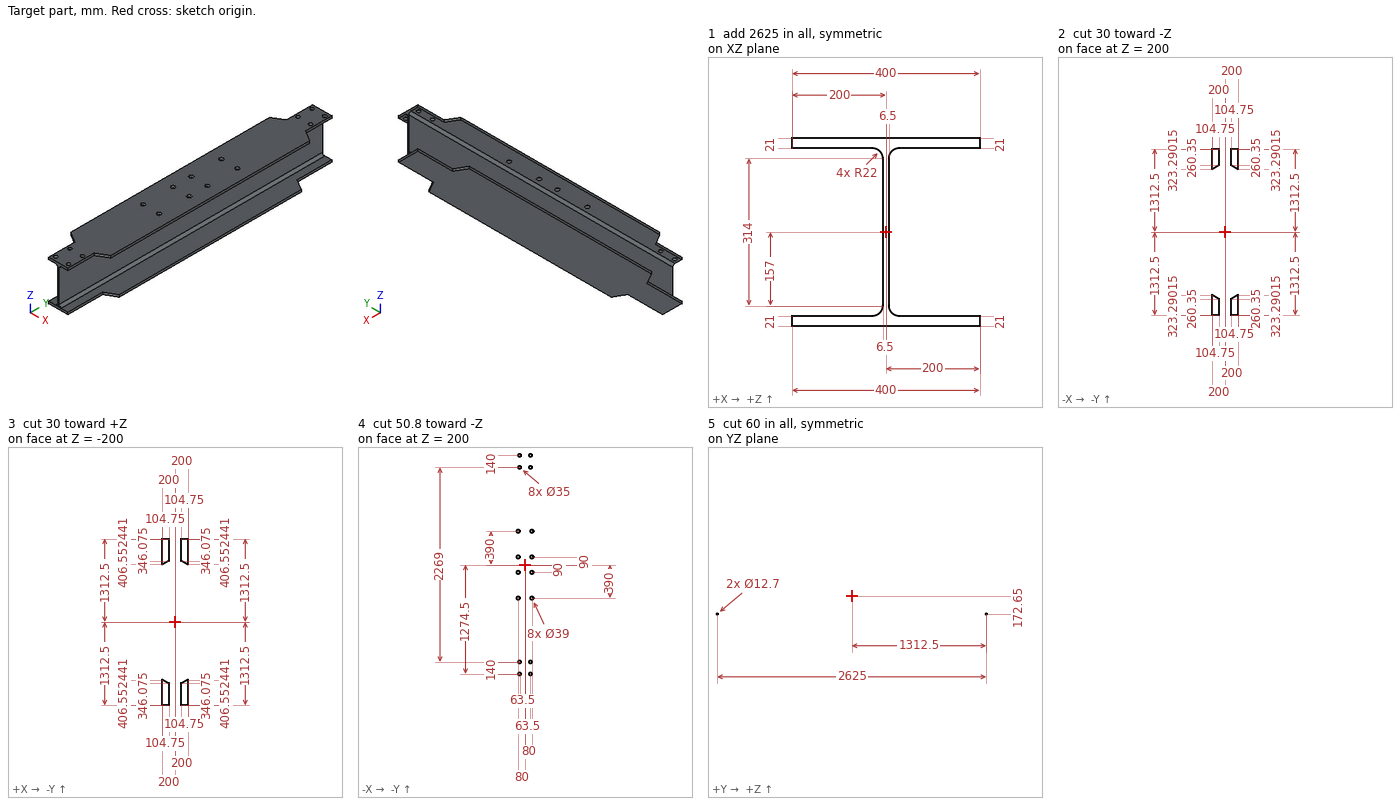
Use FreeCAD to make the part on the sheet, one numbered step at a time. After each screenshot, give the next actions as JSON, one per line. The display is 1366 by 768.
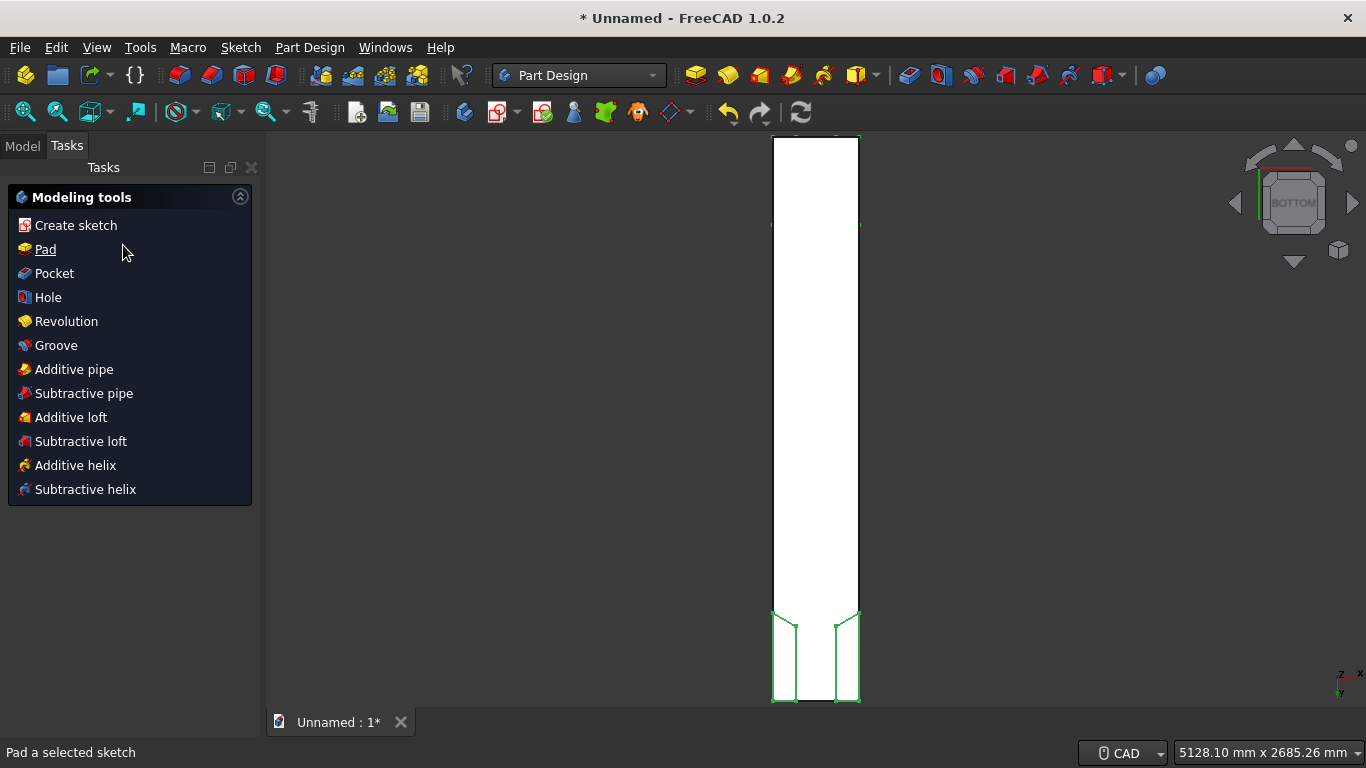
{"action": "left_click", "coordinate": [910, 76]}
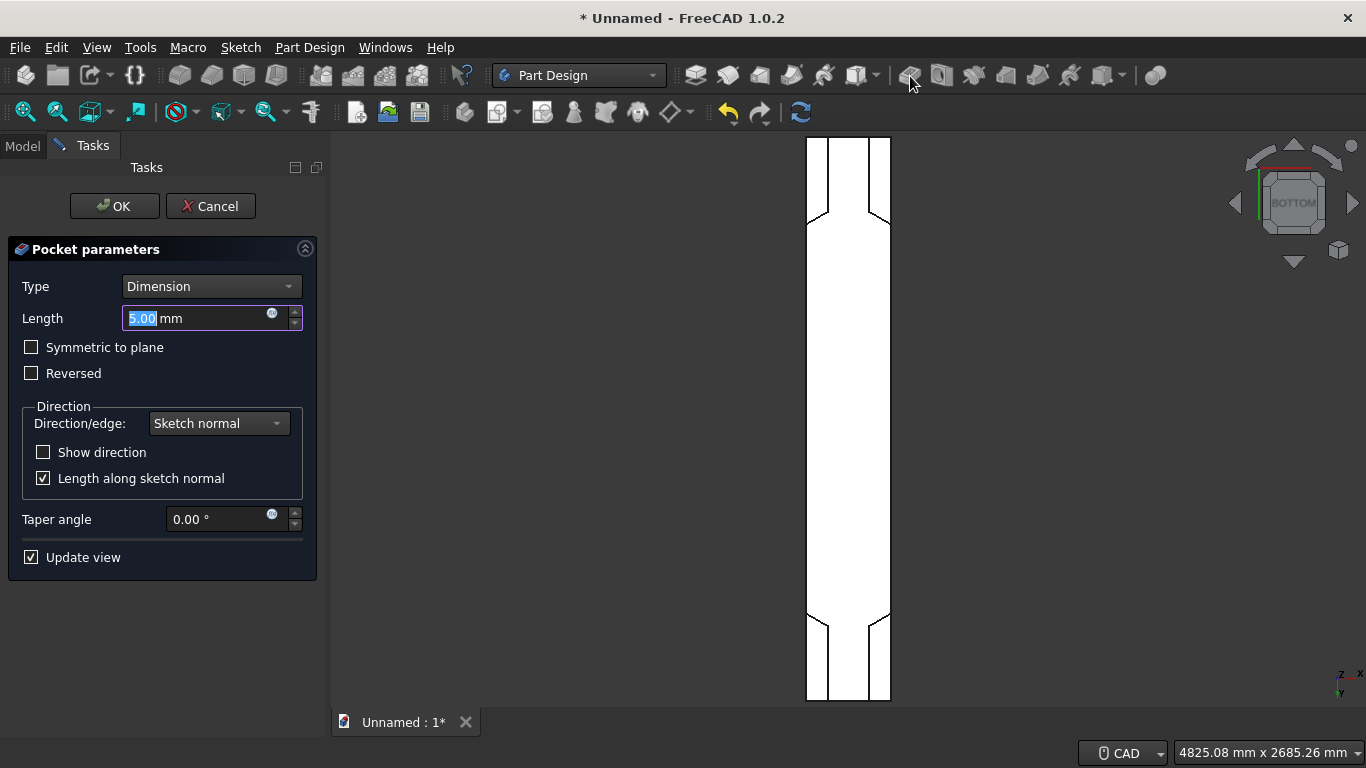
{"action": "type", "text": "30"}
{"action": "key", "text": "Tab"}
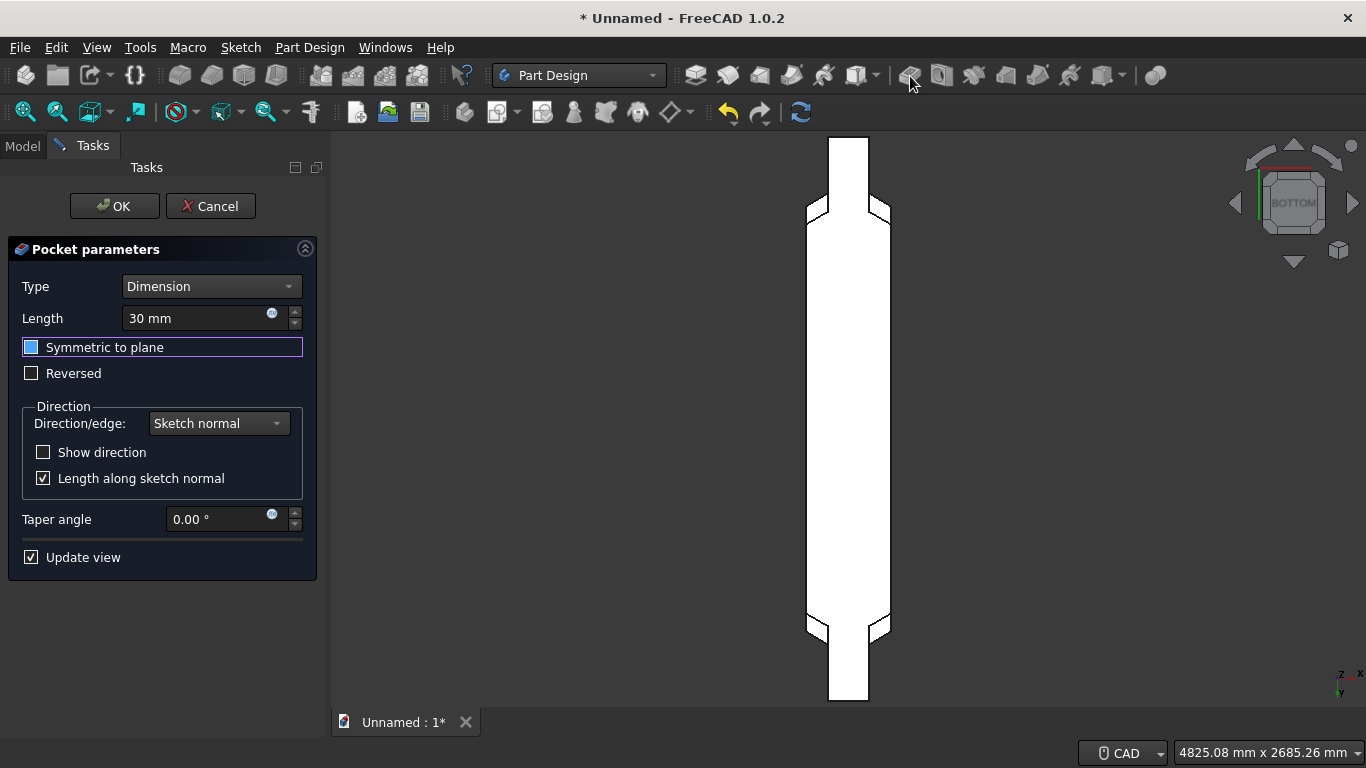
{"action": "left_click", "coordinate": [115, 206]}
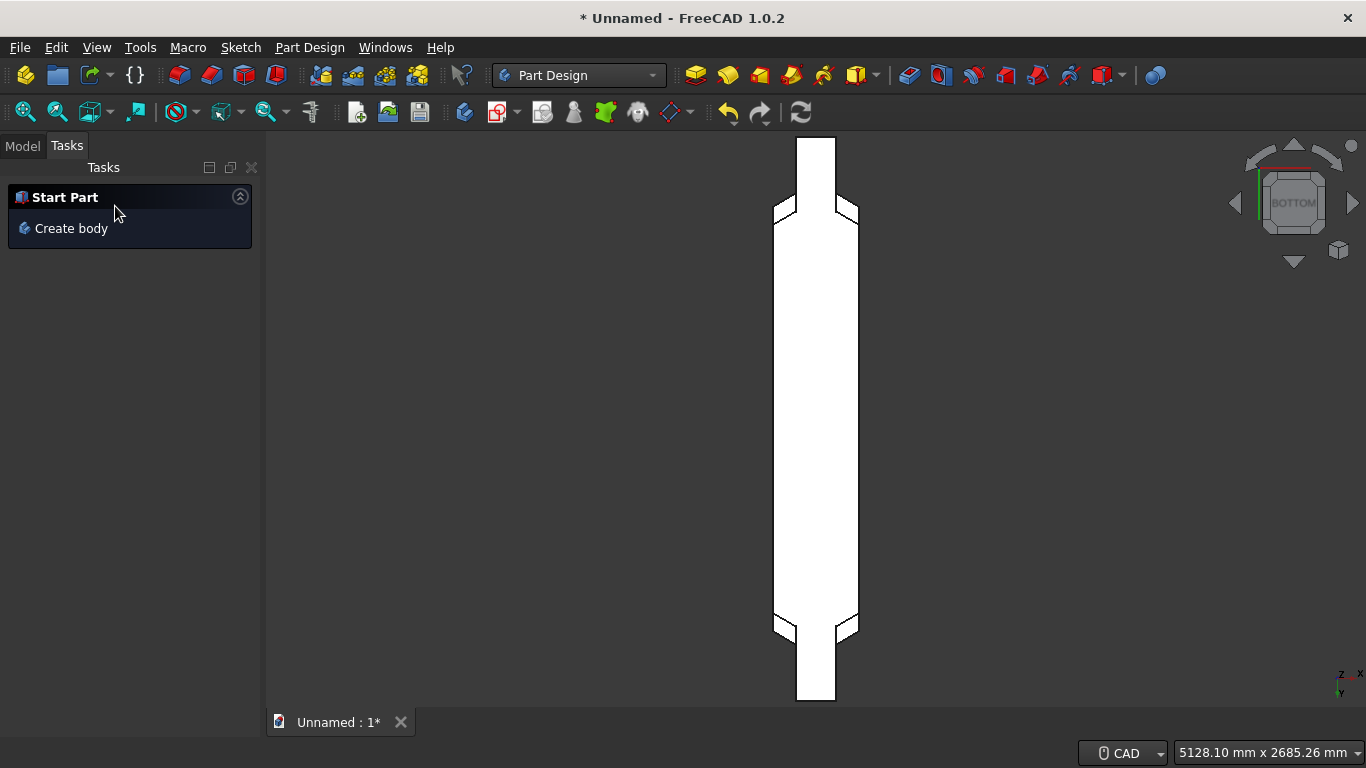
{"action": "key", "text": "0"}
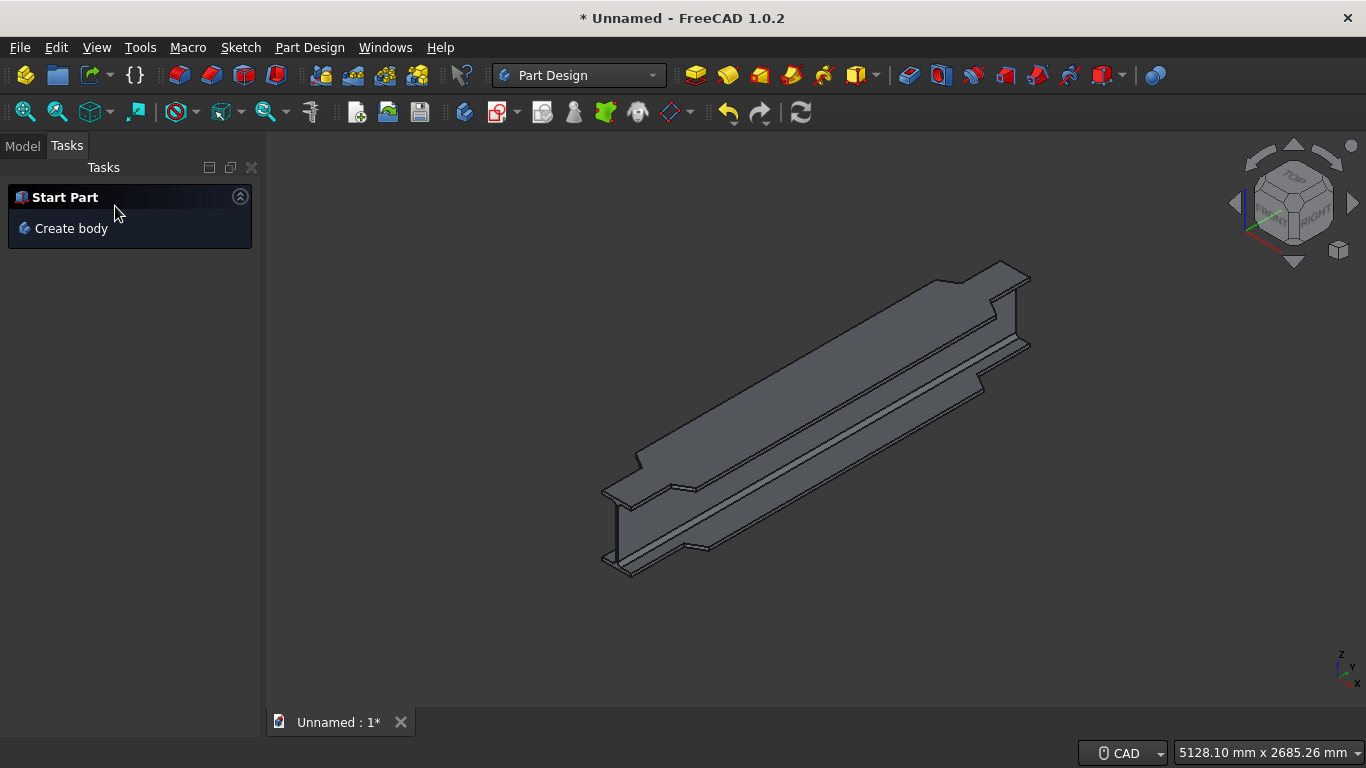
{"action": "left_click", "coordinate": [930, 317]}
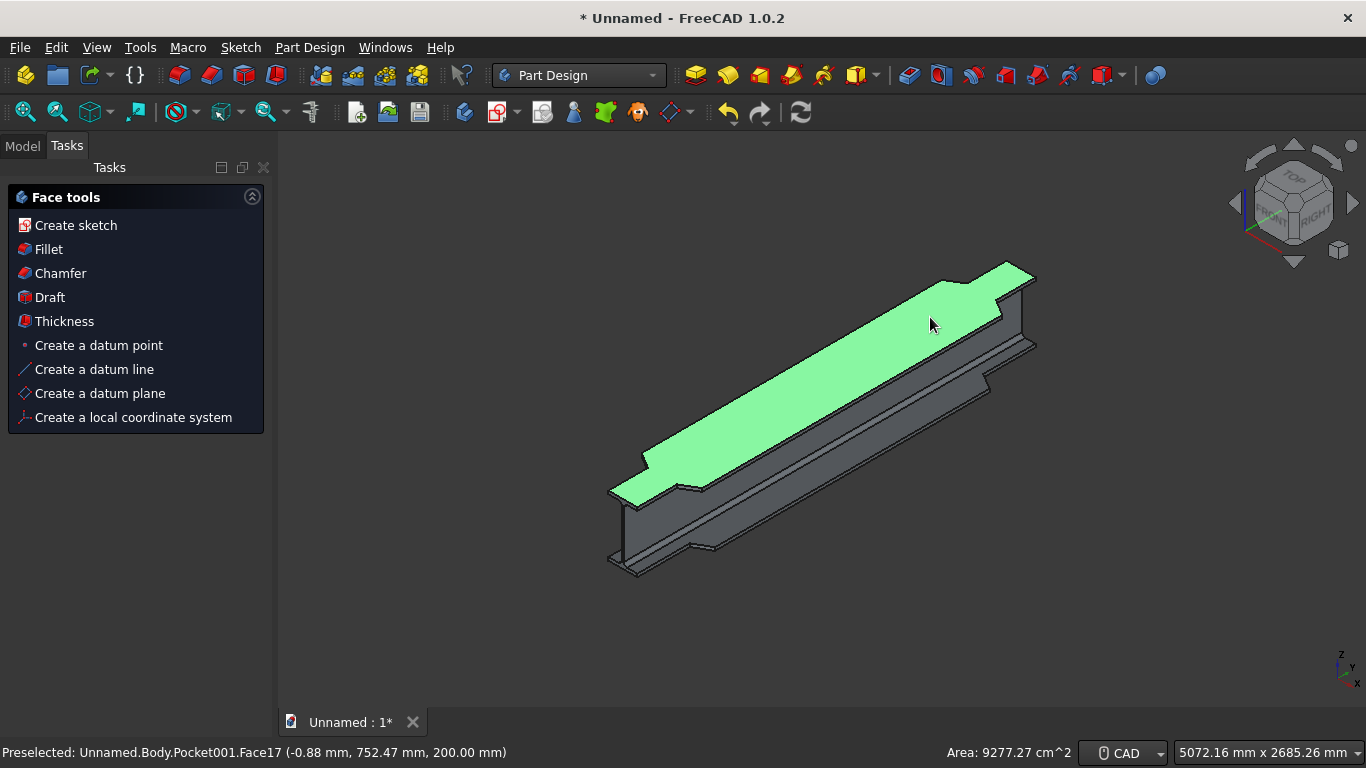
{"action": "left_click", "coordinate": [498, 112]}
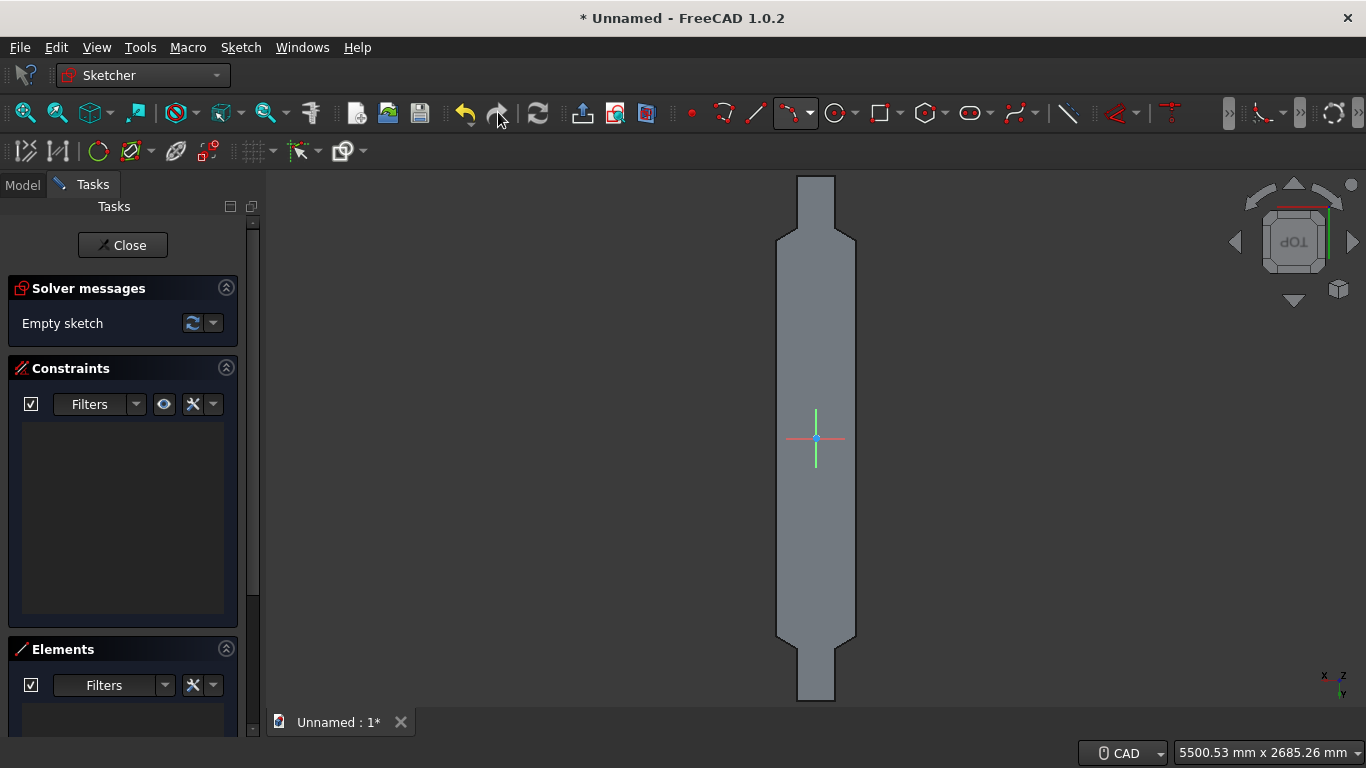
{"action": "scroll", "coordinate": [608, 438], "scroll_direction": "down", "scroll_amount": 2}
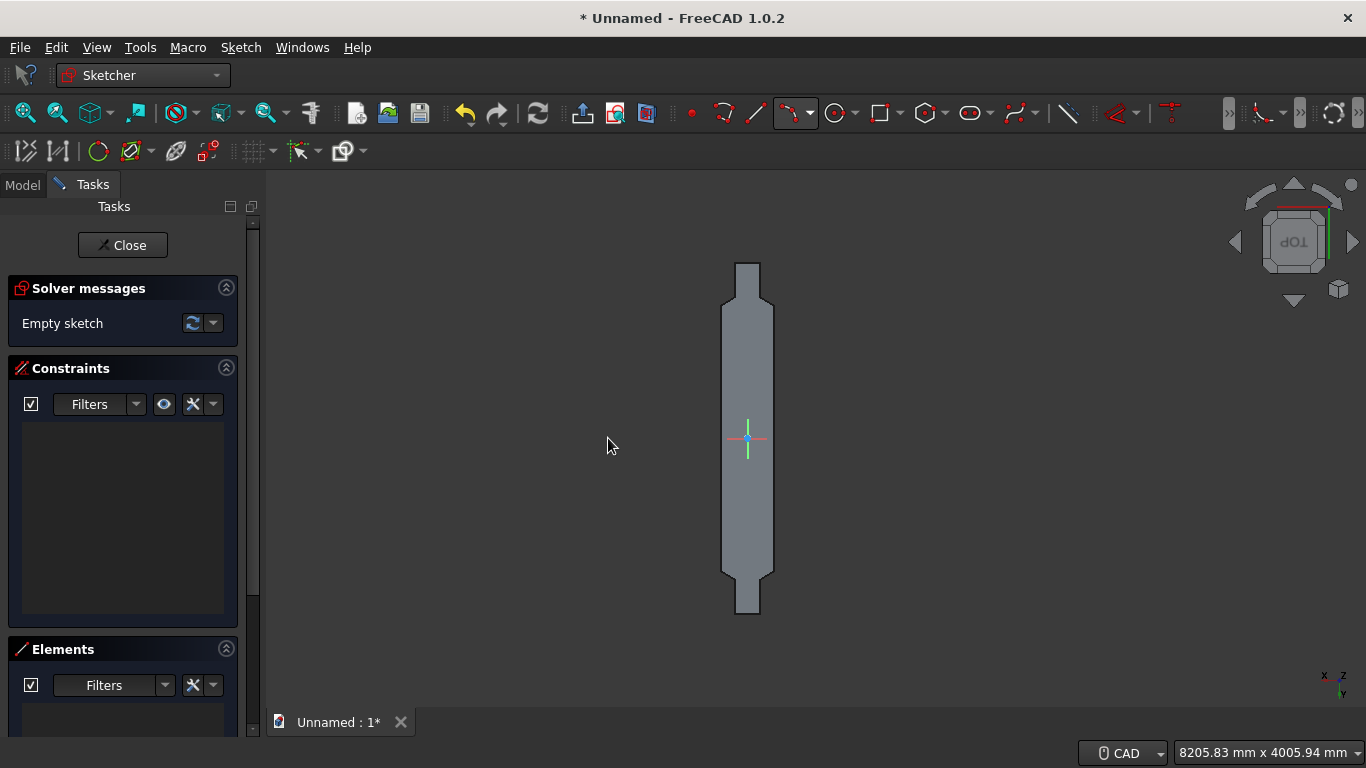
{"action": "left_click", "coordinate": [836, 114]}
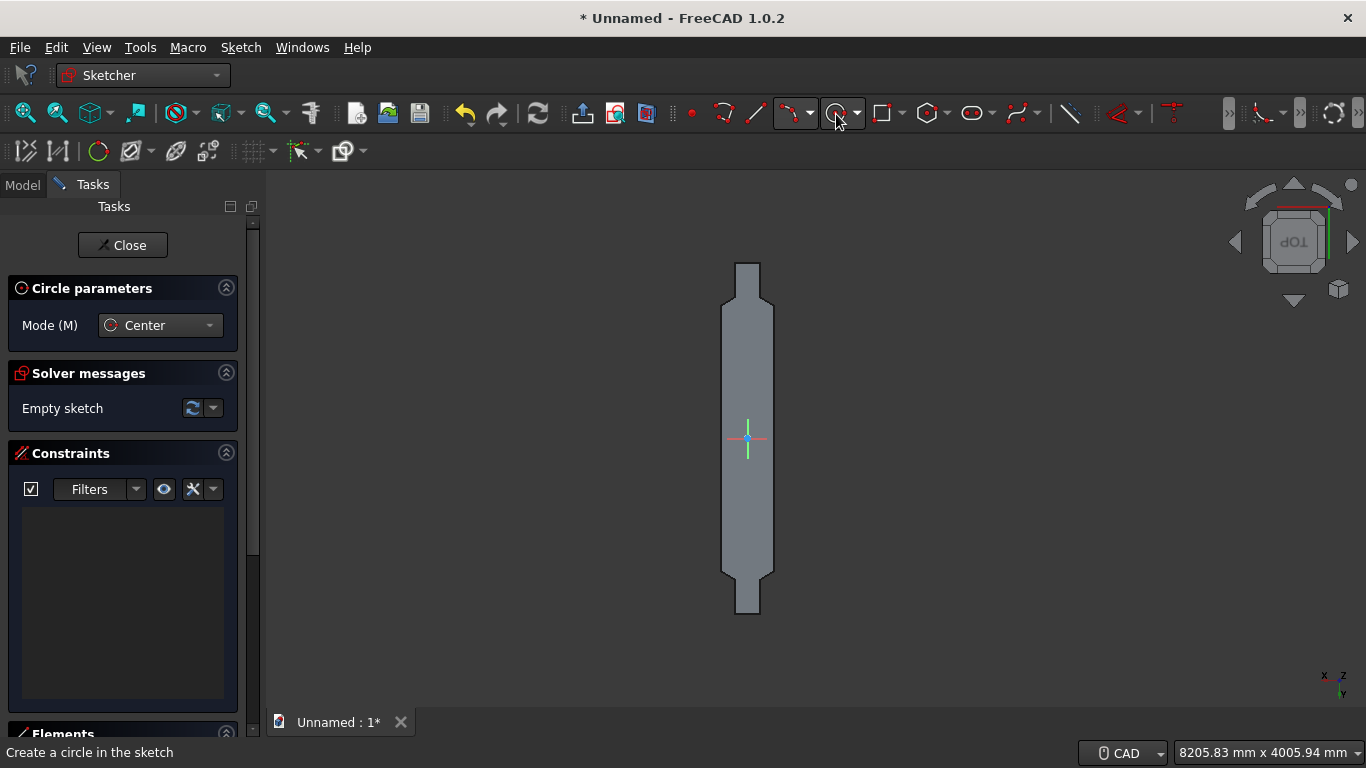
{"action": "scroll", "coordinate": [758, 491], "scroll_direction": "up", "scroll_amount": 11}